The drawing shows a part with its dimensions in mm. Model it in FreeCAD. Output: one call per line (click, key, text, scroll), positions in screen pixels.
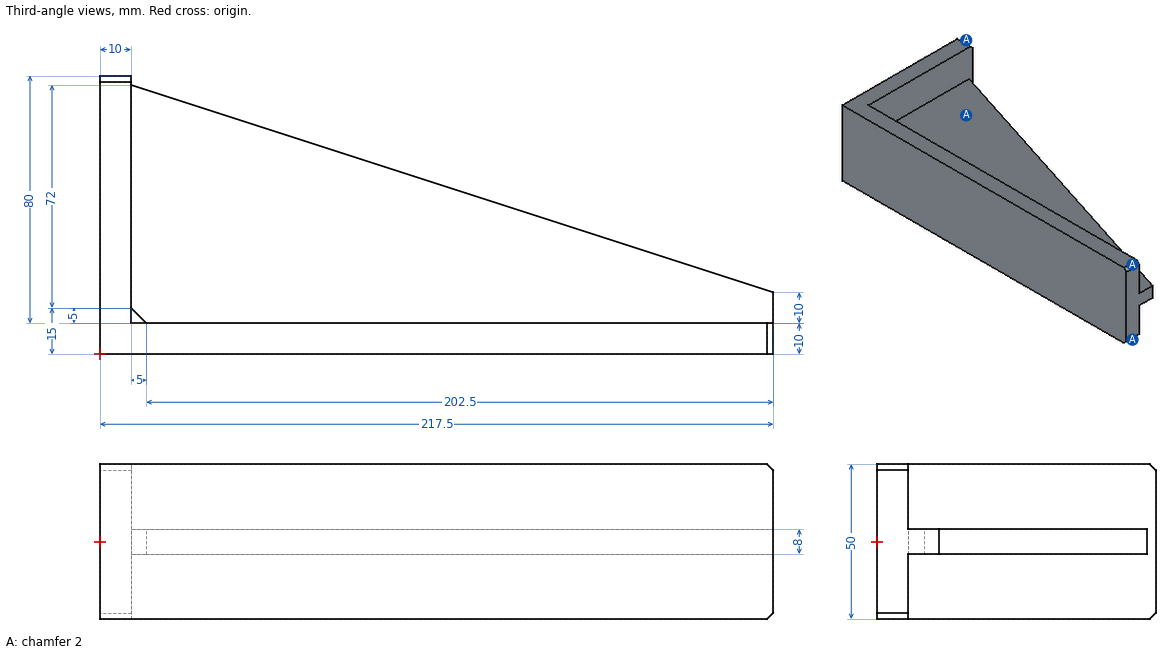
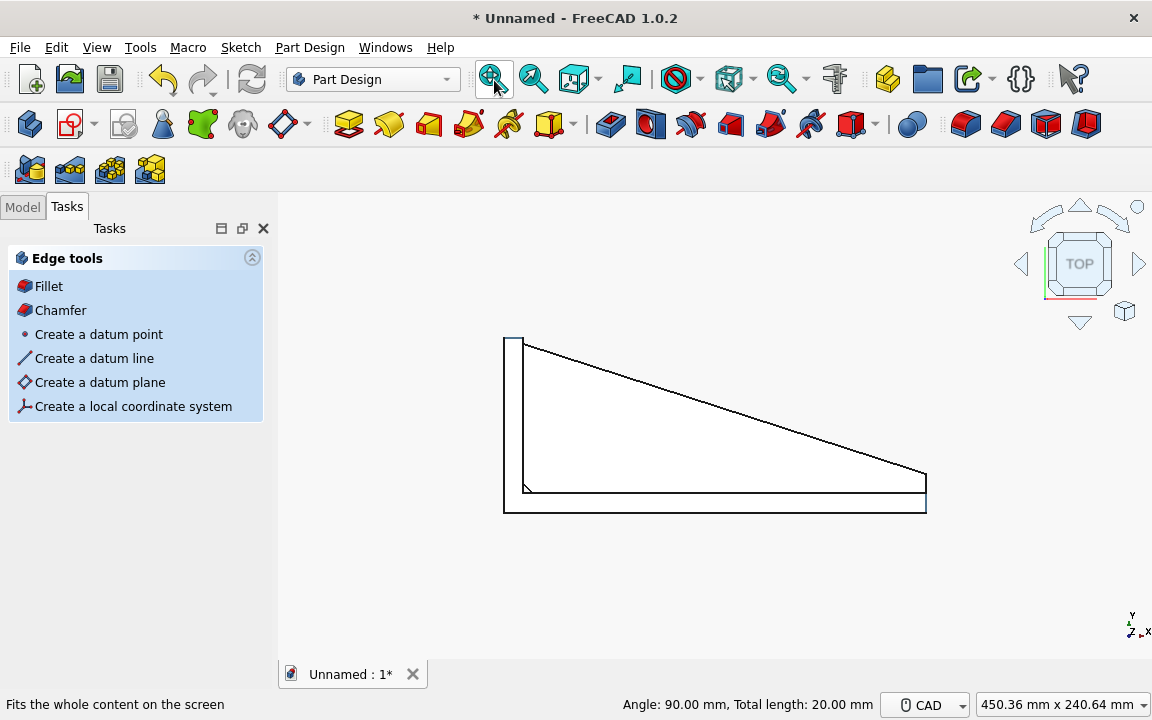
key(1)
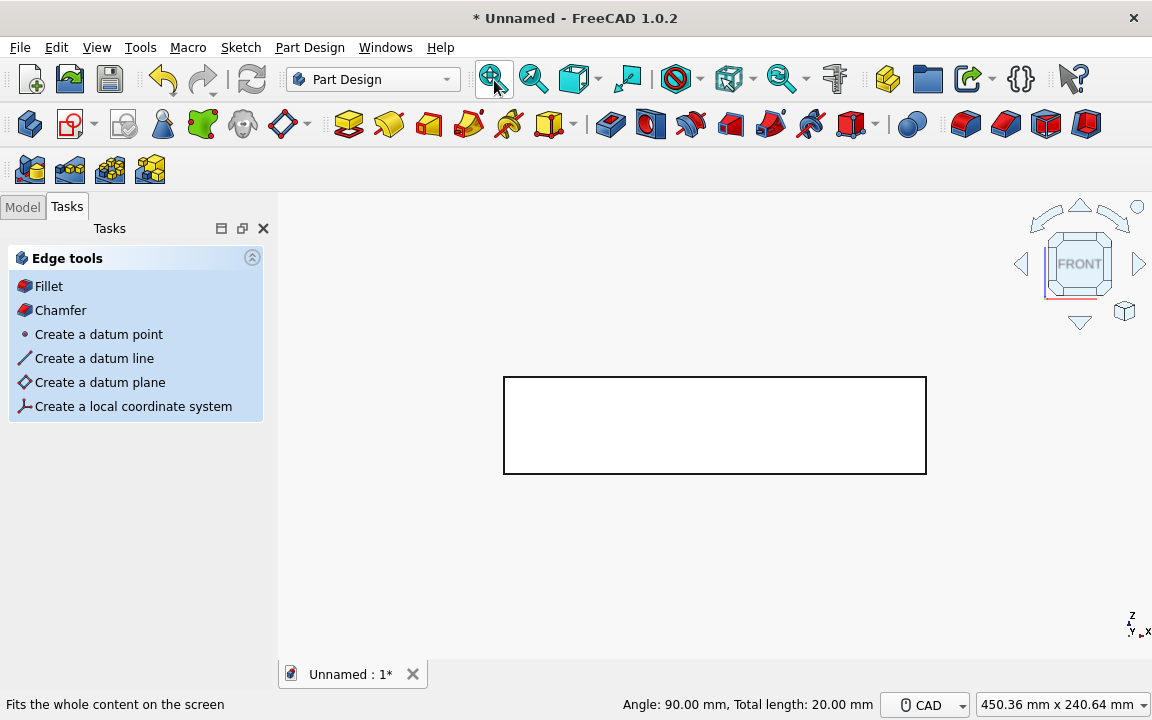
scroll(514, 473, up, 4)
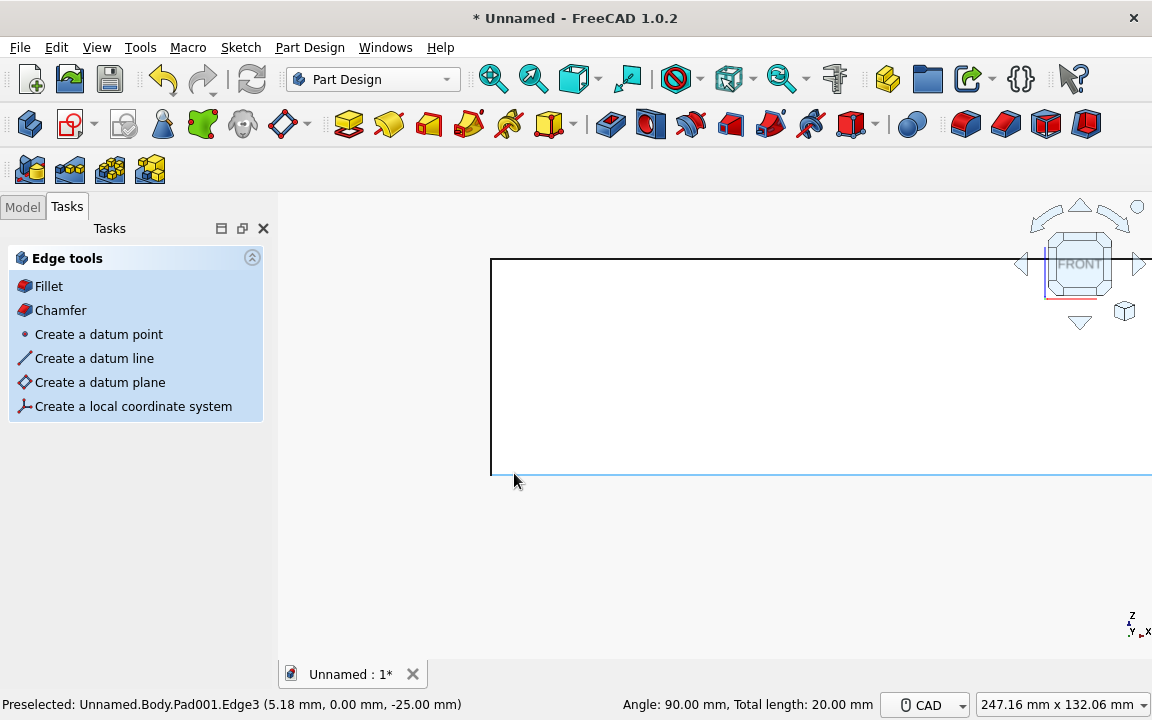
click(494, 80)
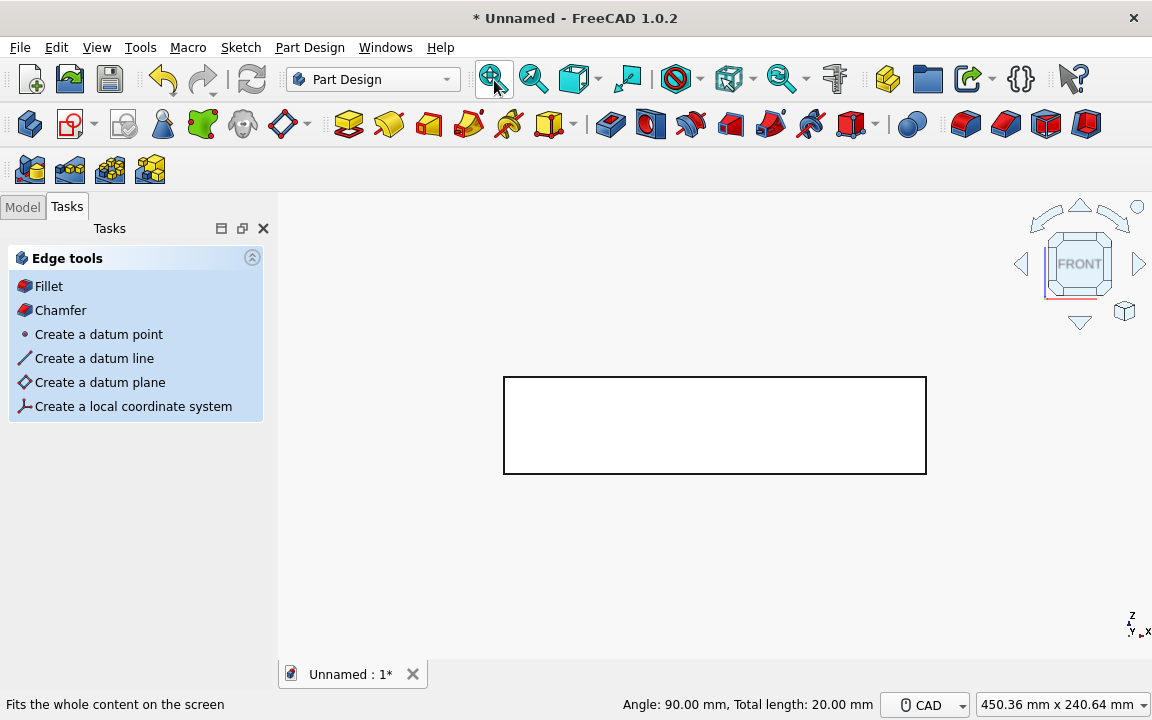
key(3)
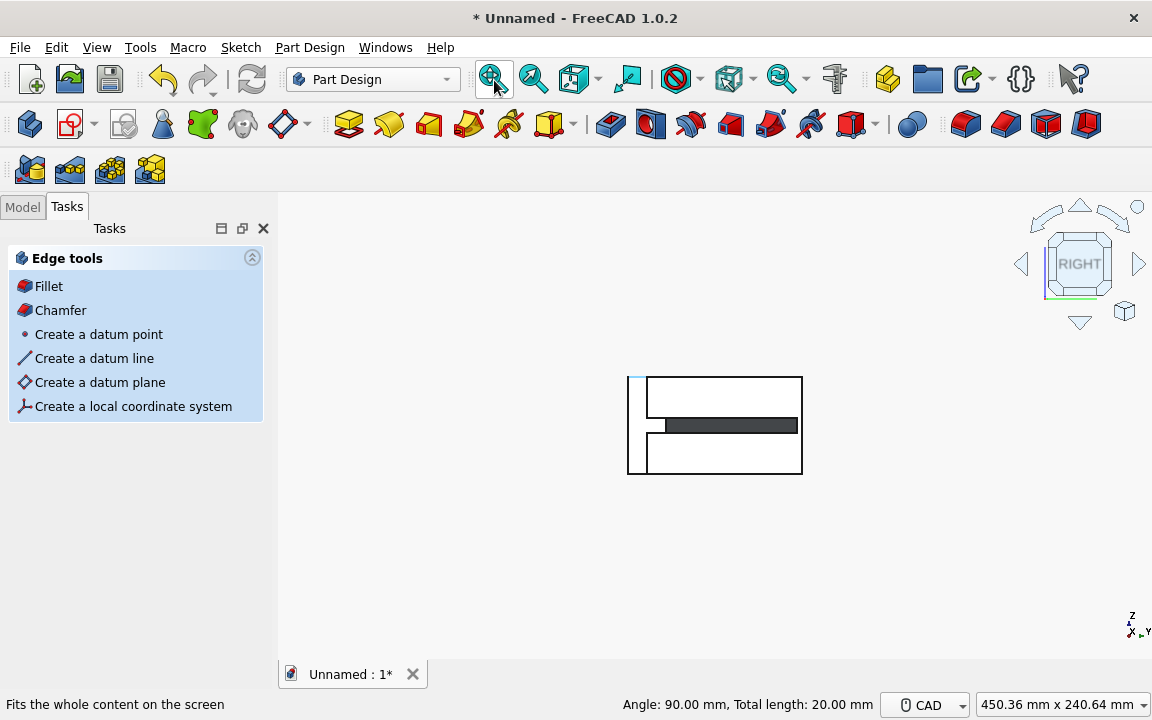
click(494, 80)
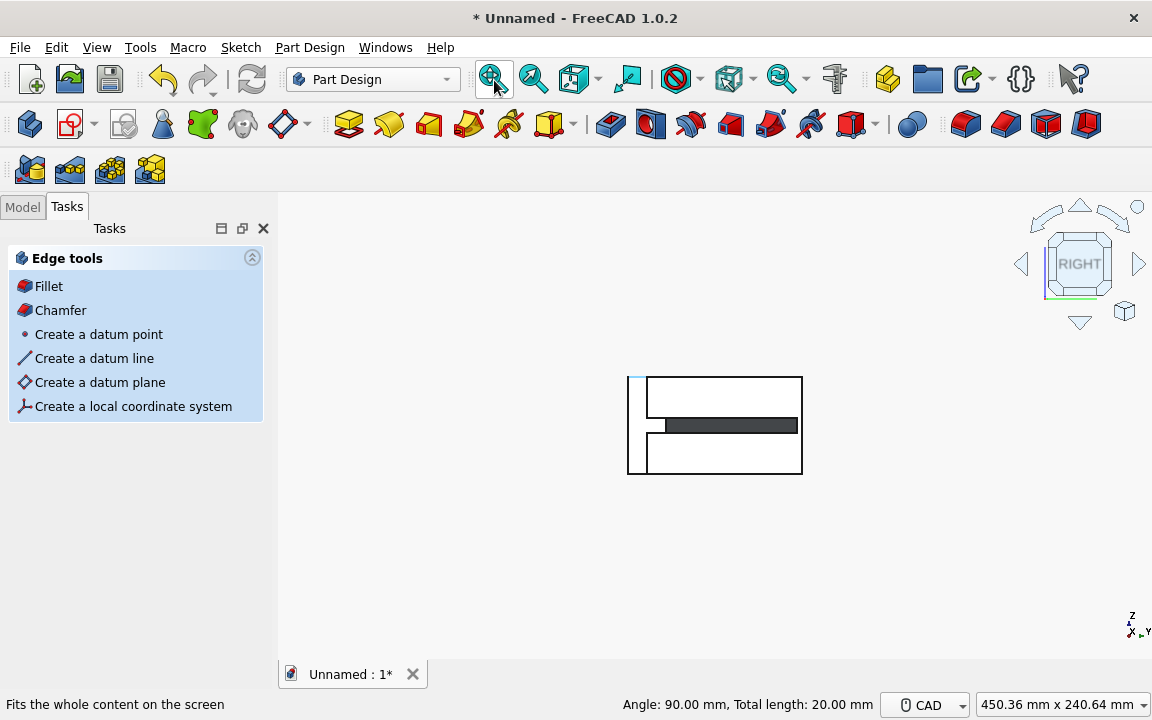
click(637, 473, ctrl)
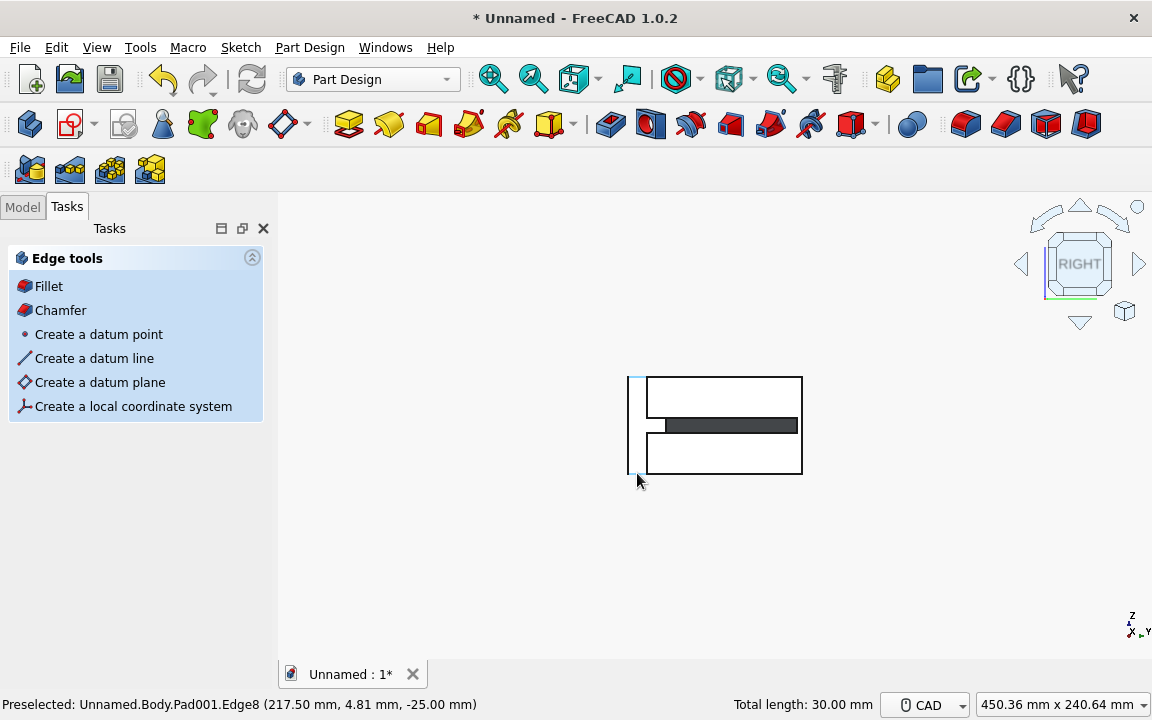
scroll(802, 473, up, 4)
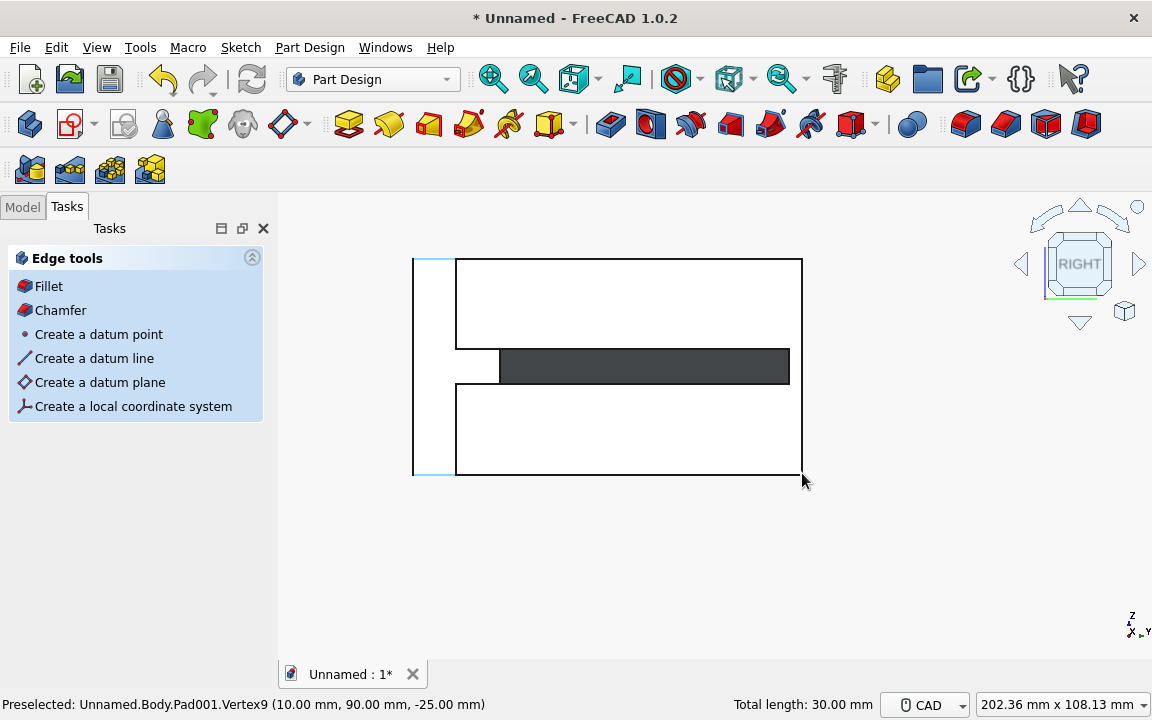
click(494, 80)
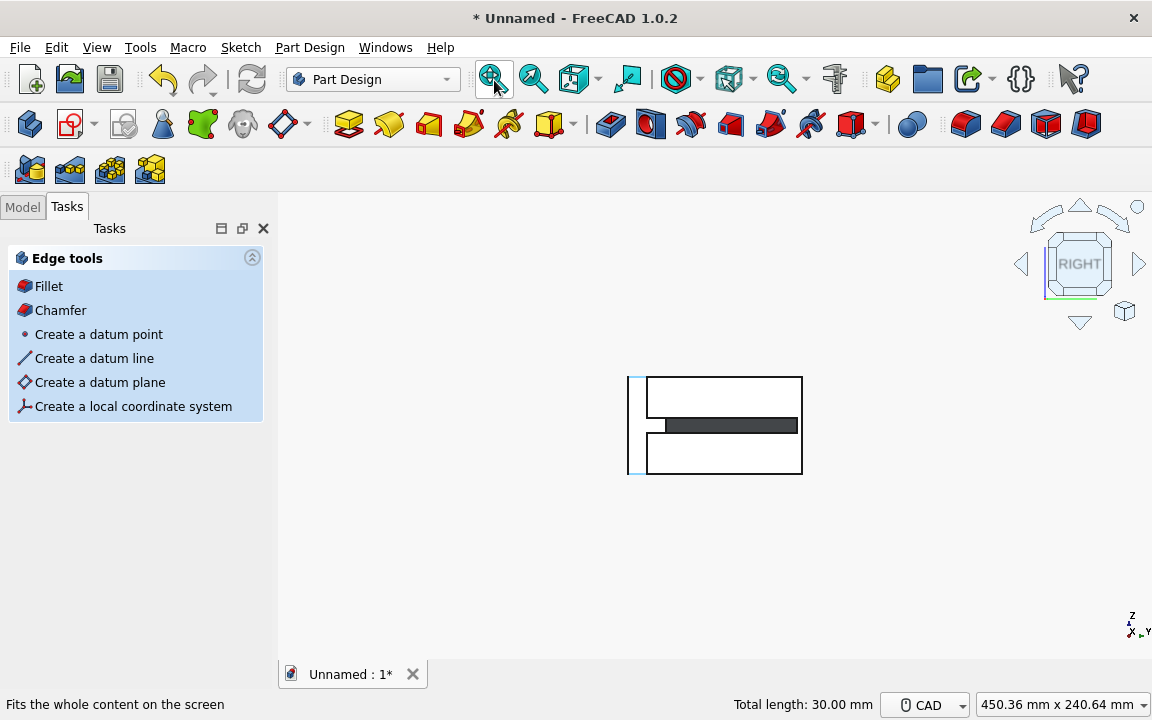
key(5)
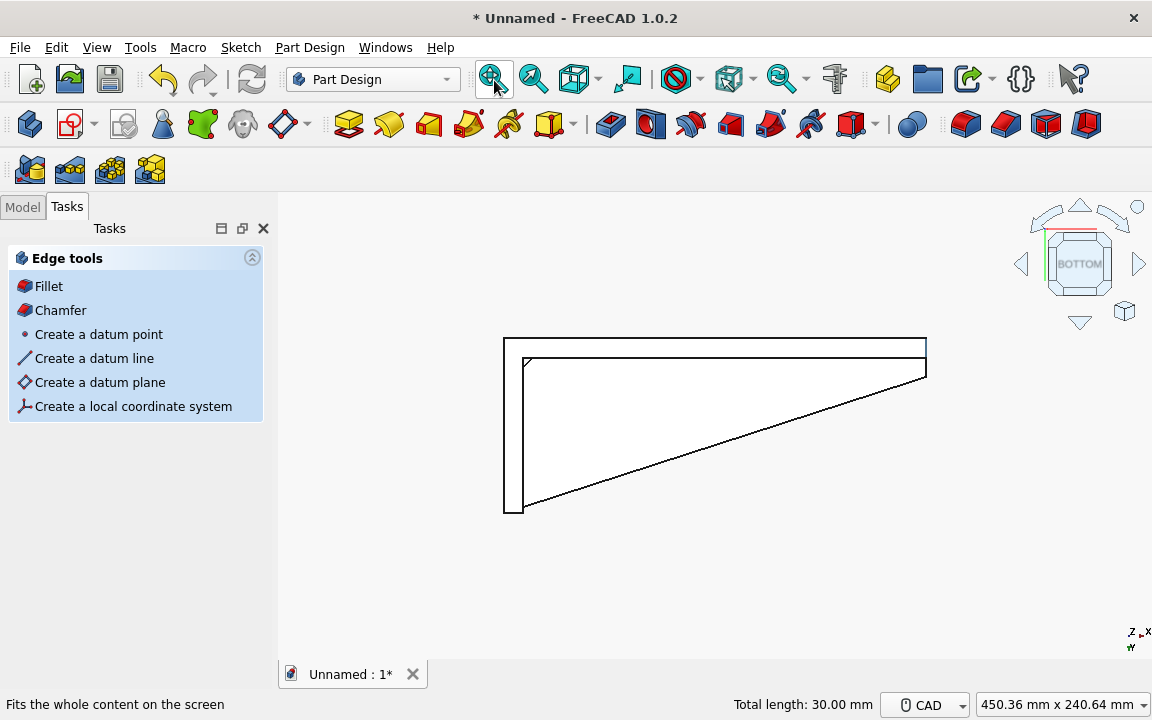
click(514, 512, ctrl)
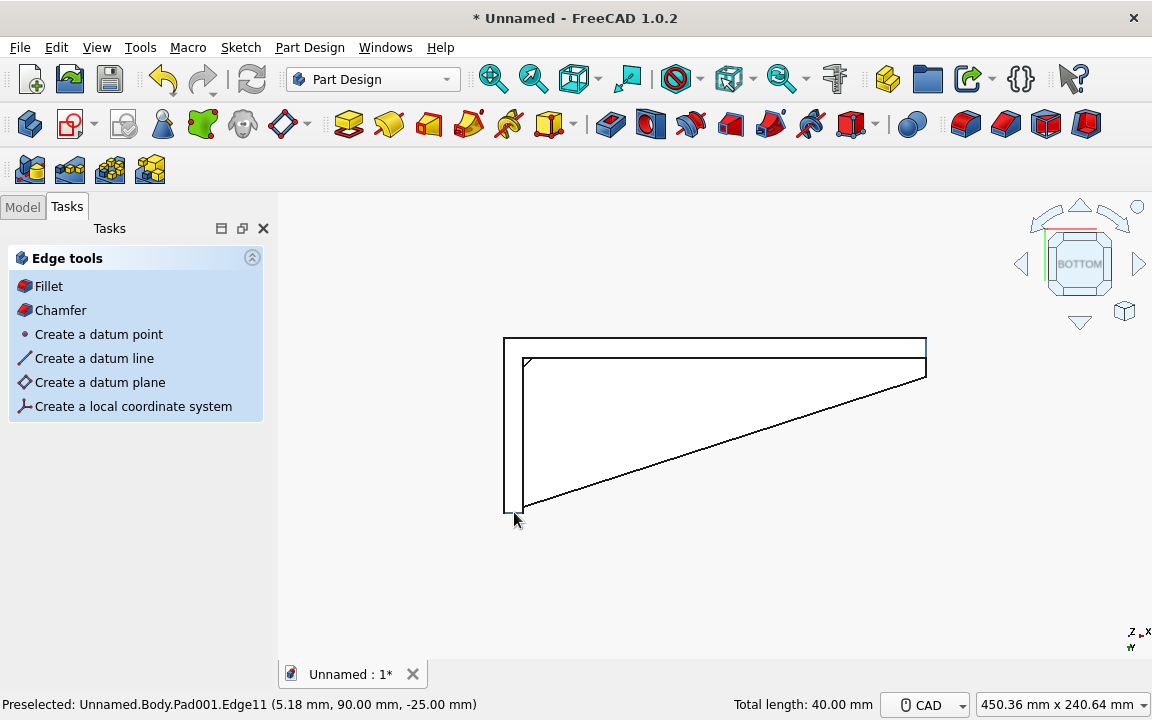
click(1006, 124)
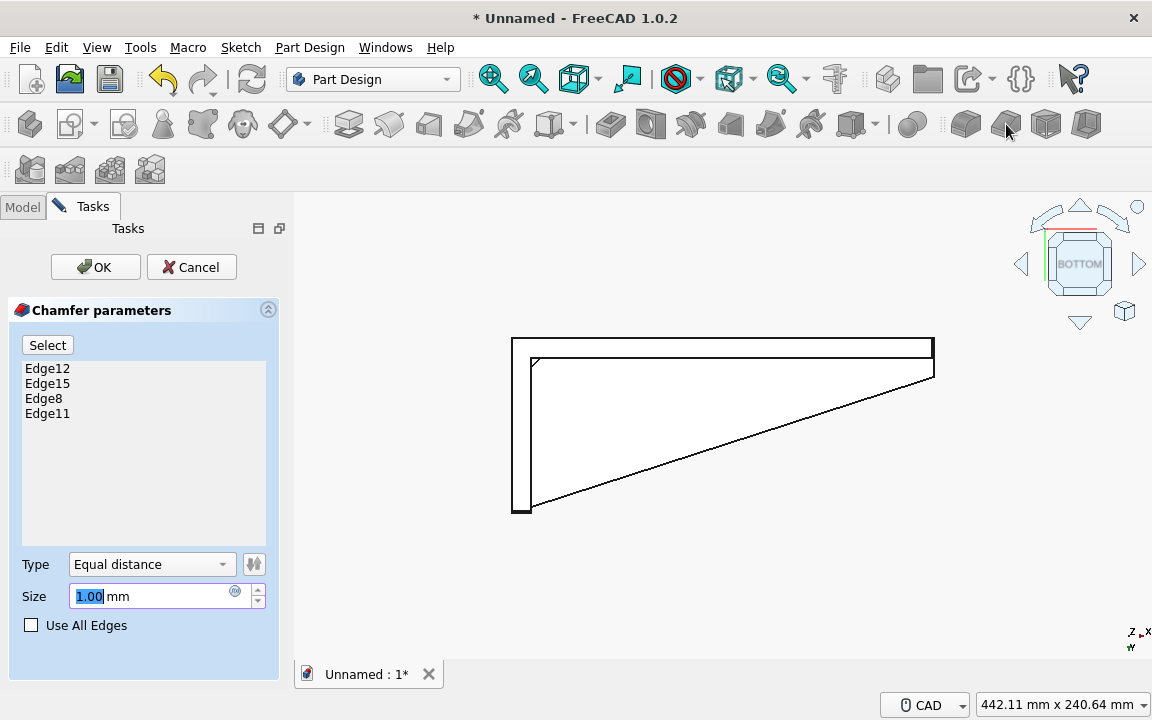
text(2)
key(Tab)